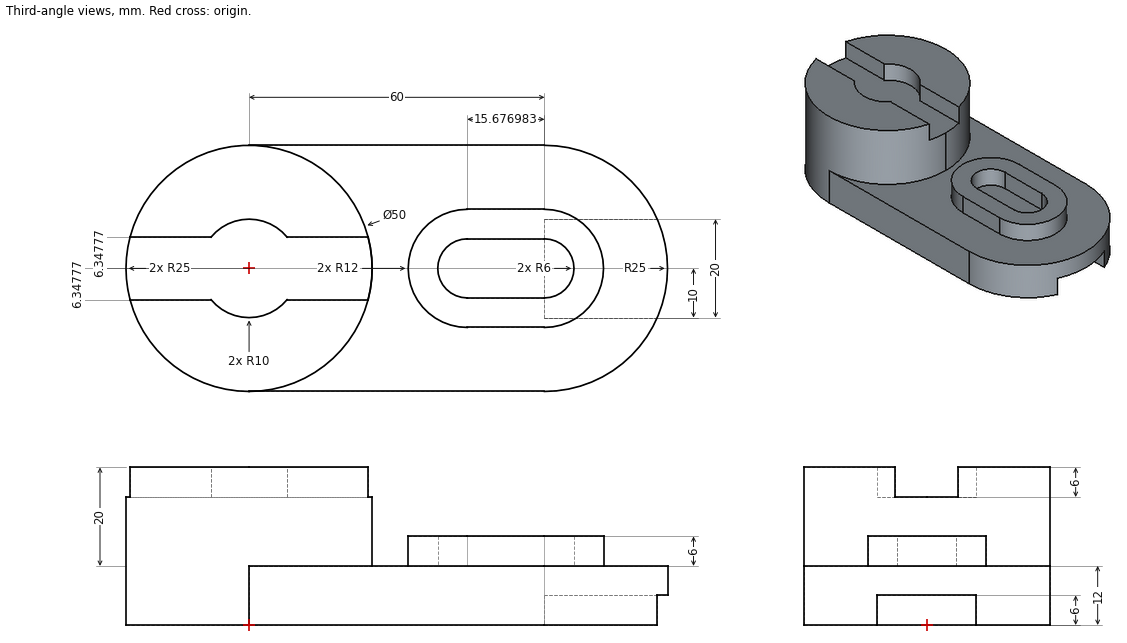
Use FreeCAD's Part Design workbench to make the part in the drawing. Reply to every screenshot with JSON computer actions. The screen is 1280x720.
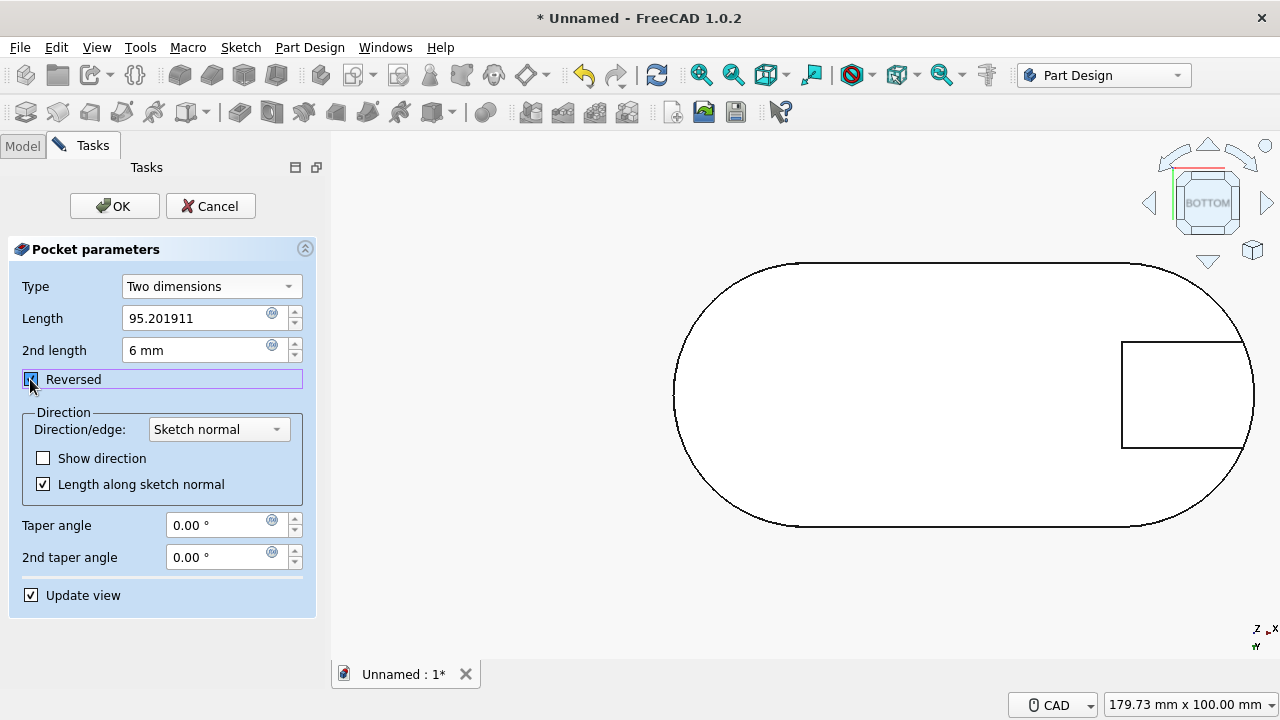
{"action": "left_click", "coordinate": [115, 206]}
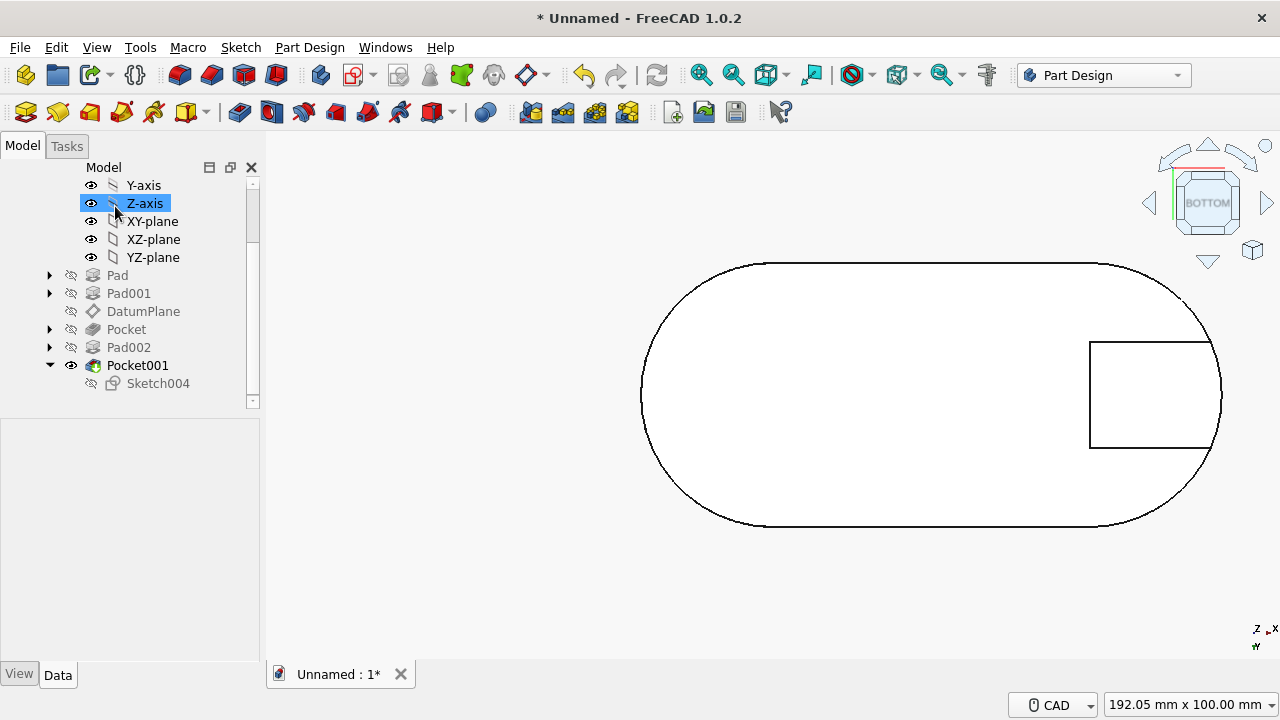
{"action": "key", "text": "0"}